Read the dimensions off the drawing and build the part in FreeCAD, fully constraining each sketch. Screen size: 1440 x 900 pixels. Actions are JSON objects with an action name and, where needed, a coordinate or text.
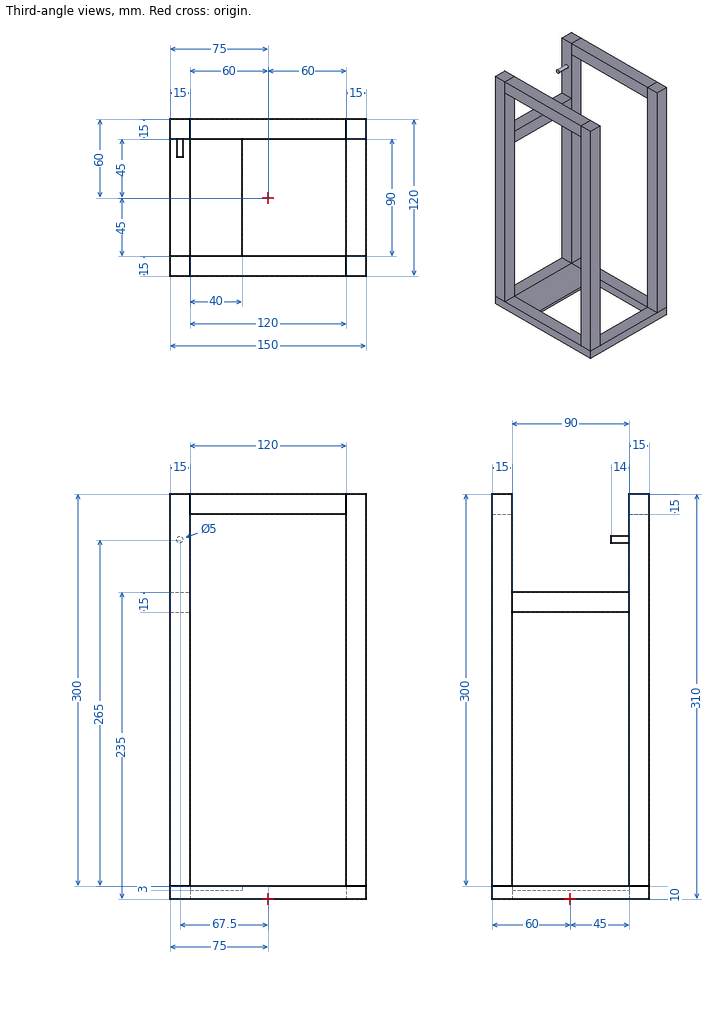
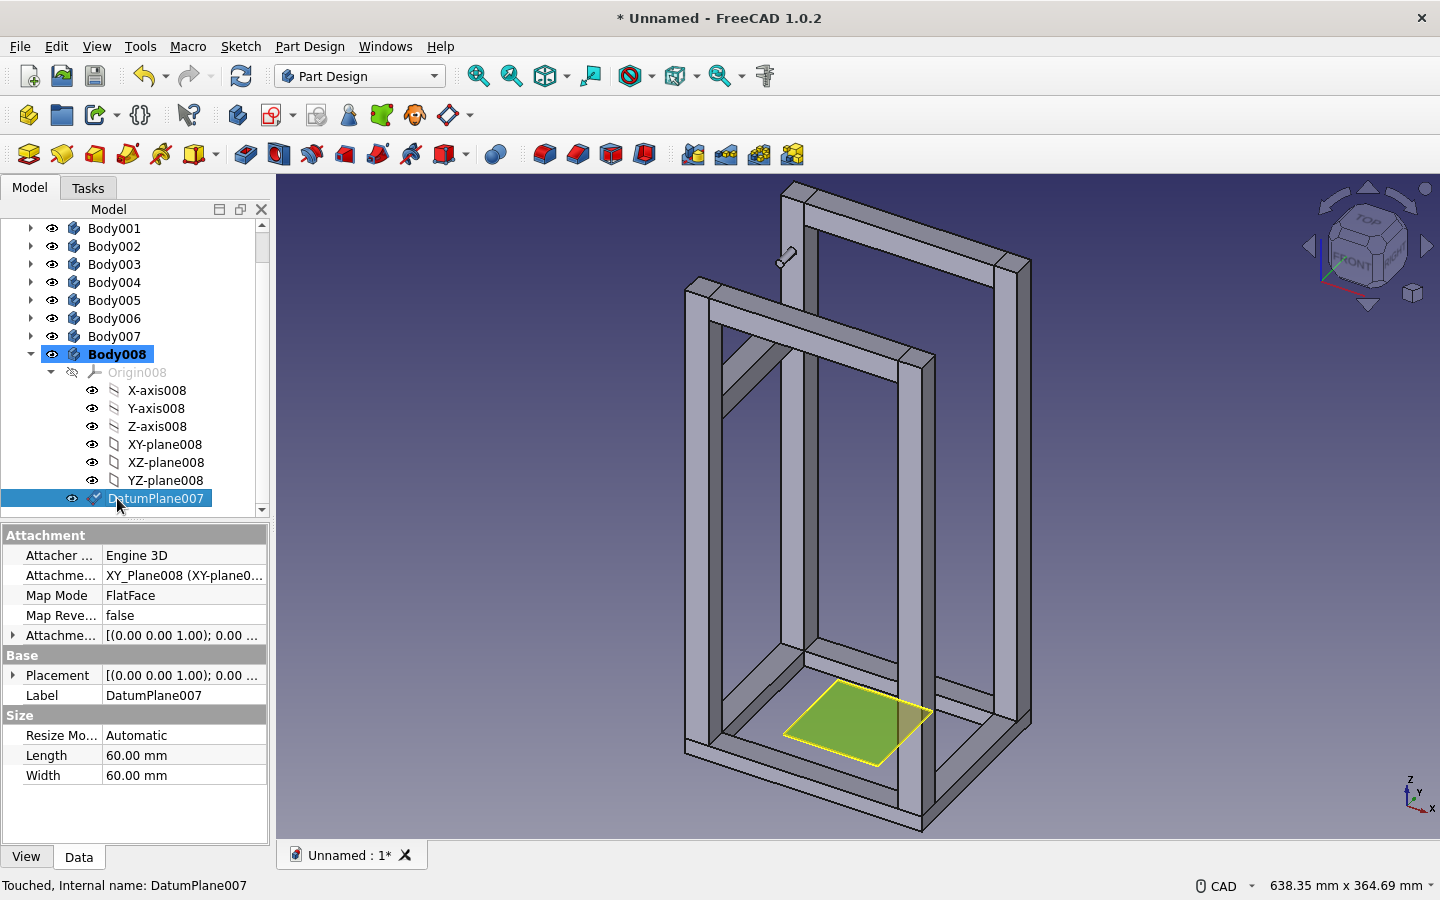
{"action": "left_click", "coordinate": [270, 116]}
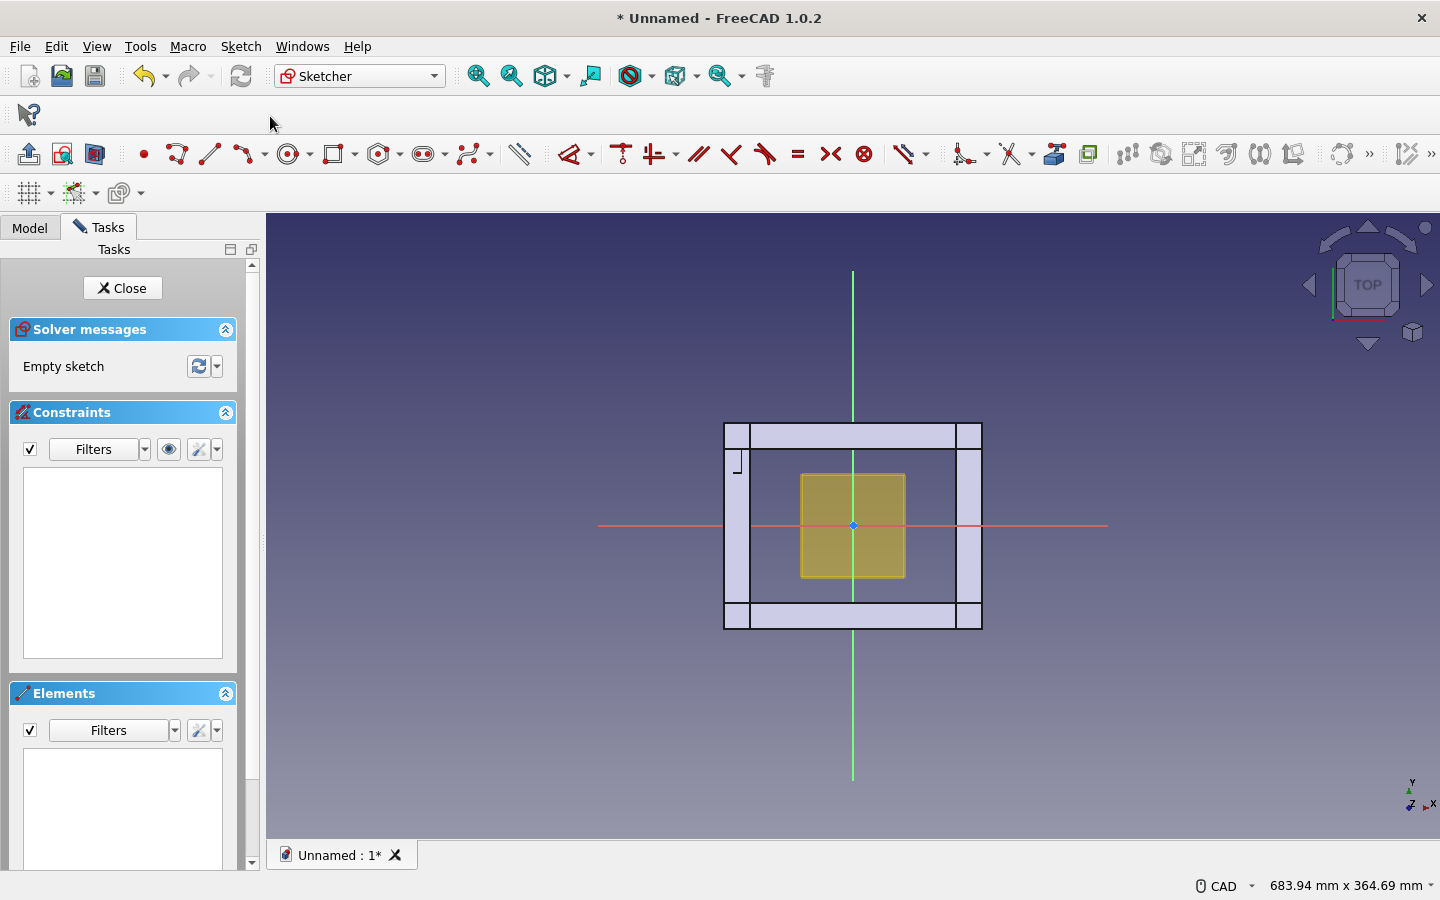
{"action": "scroll", "coordinate": [811, 526], "scroll_direction": "up", "scroll_amount": 5}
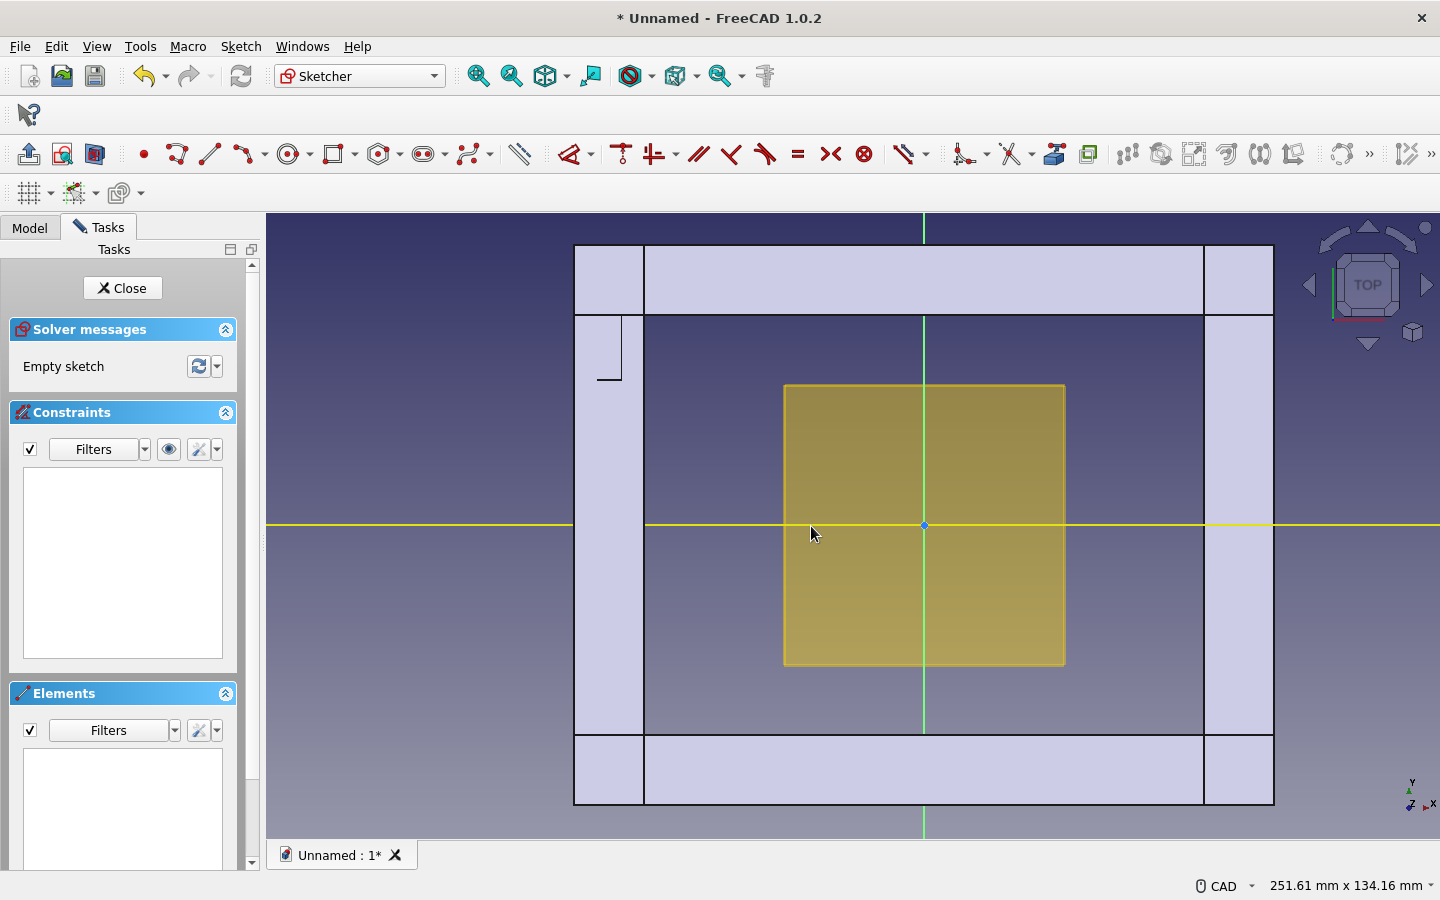
{"action": "left_click", "coordinate": [332, 154]}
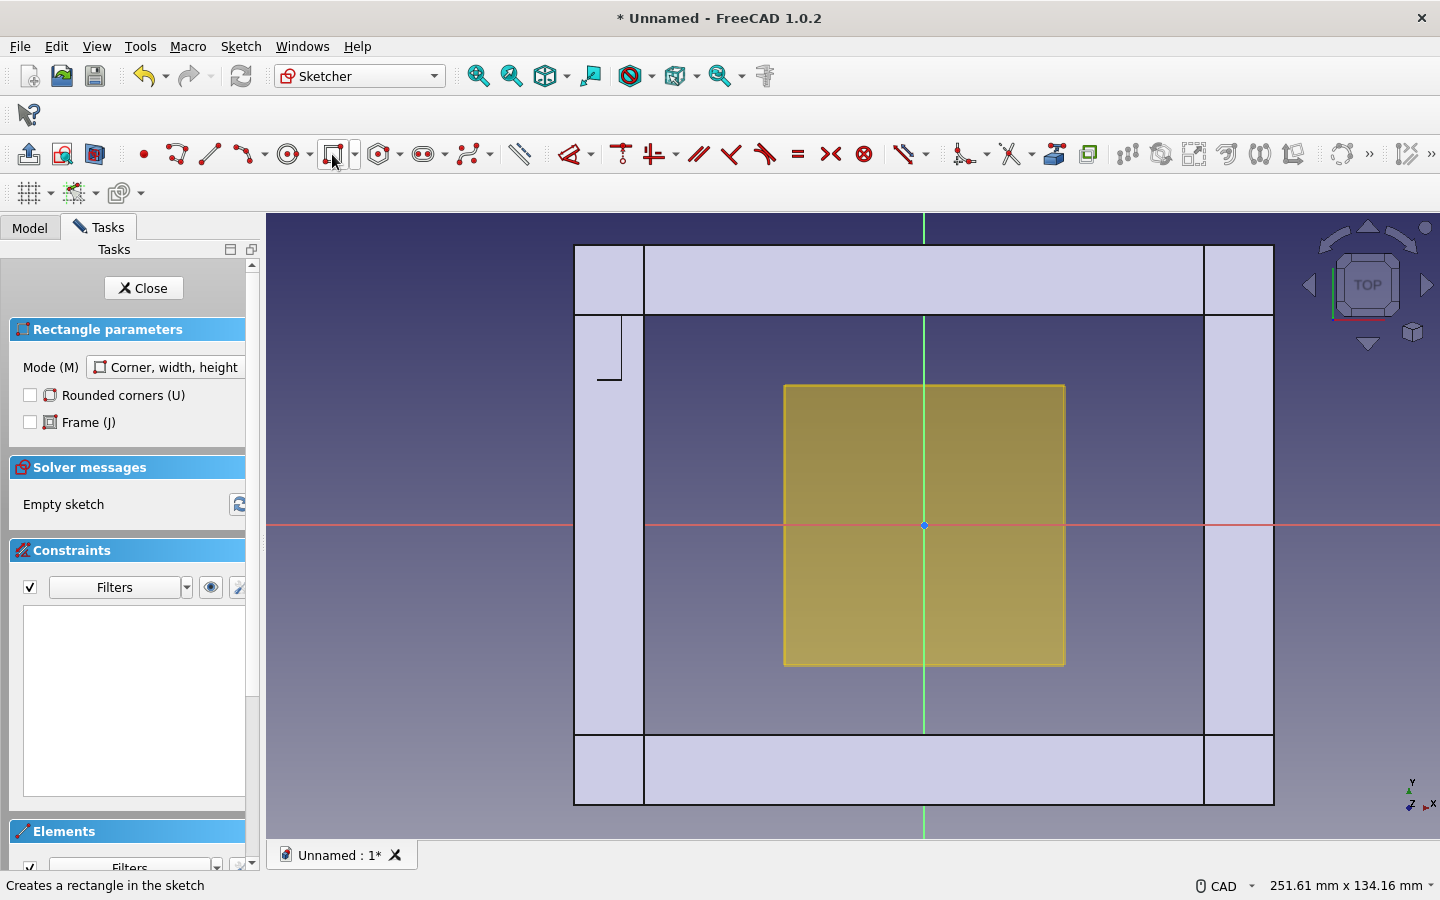
{"action": "left_click", "coordinate": [644, 315]}
{"action": "left_click", "coordinate": [831, 735]}
{"action": "key", "text": "Escape"}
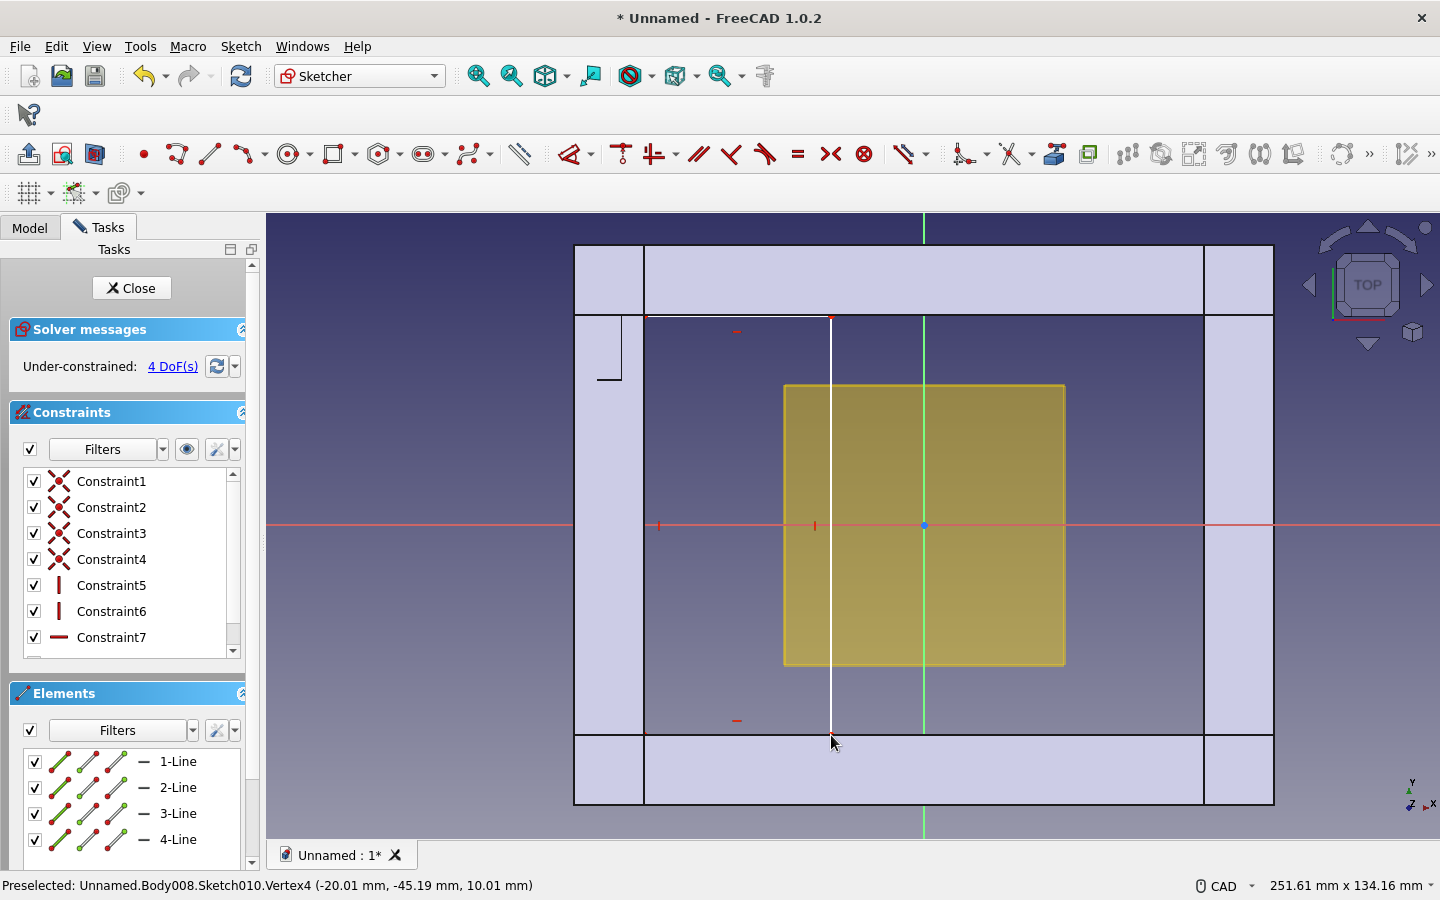
{"action": "left_click", "coordinate": [568, 154]}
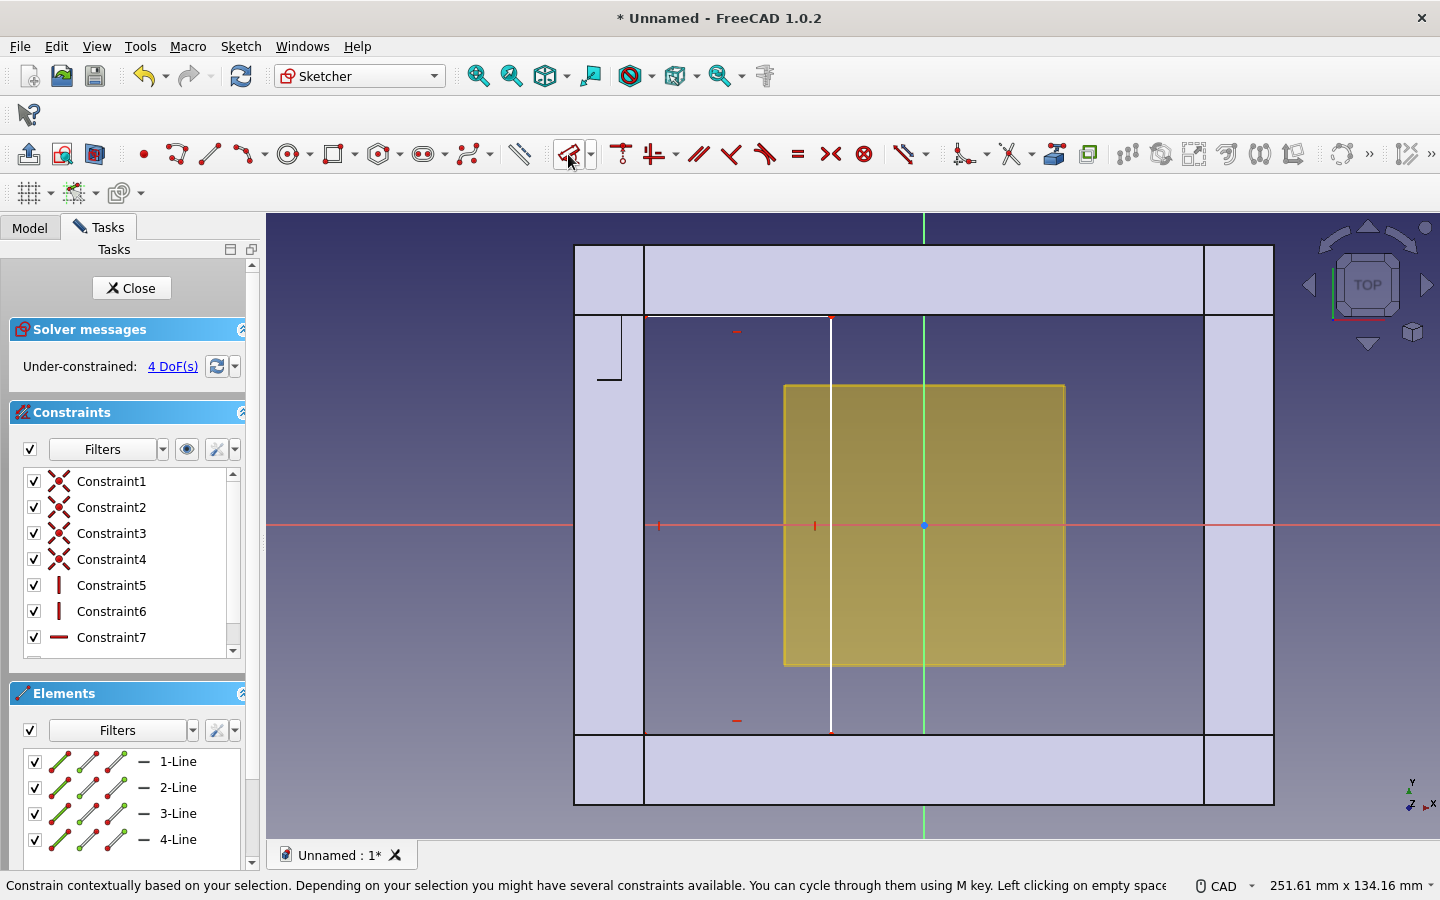
{"action": "left_click", "coordinate": [644, 442]}
{"action": "left_click", "coordinate": [610, 429]}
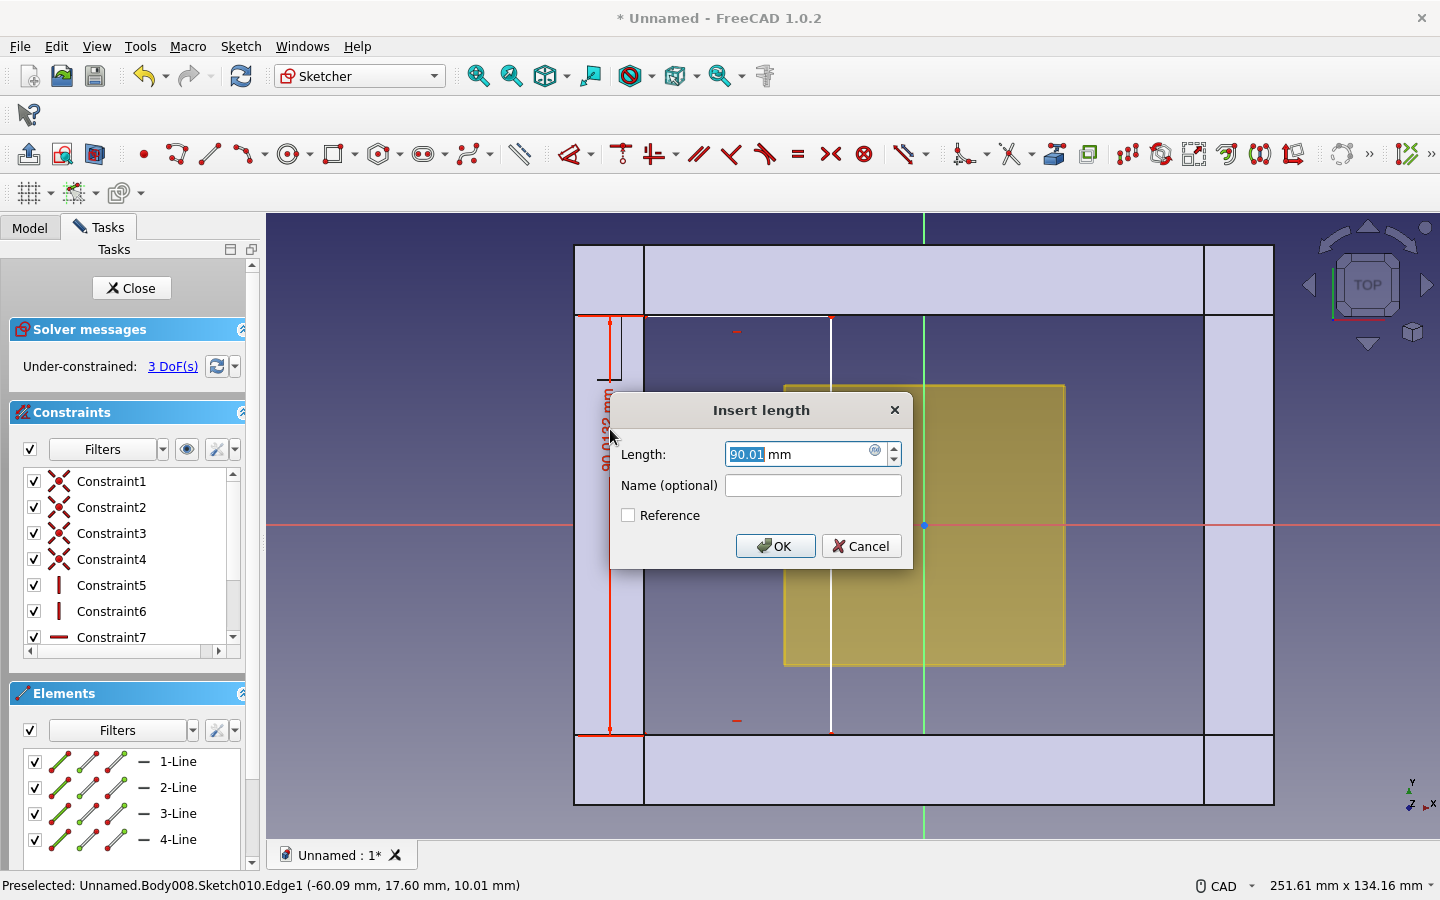
{"action": "type", "text": "90"}
{"action": "key", "text": "Return"}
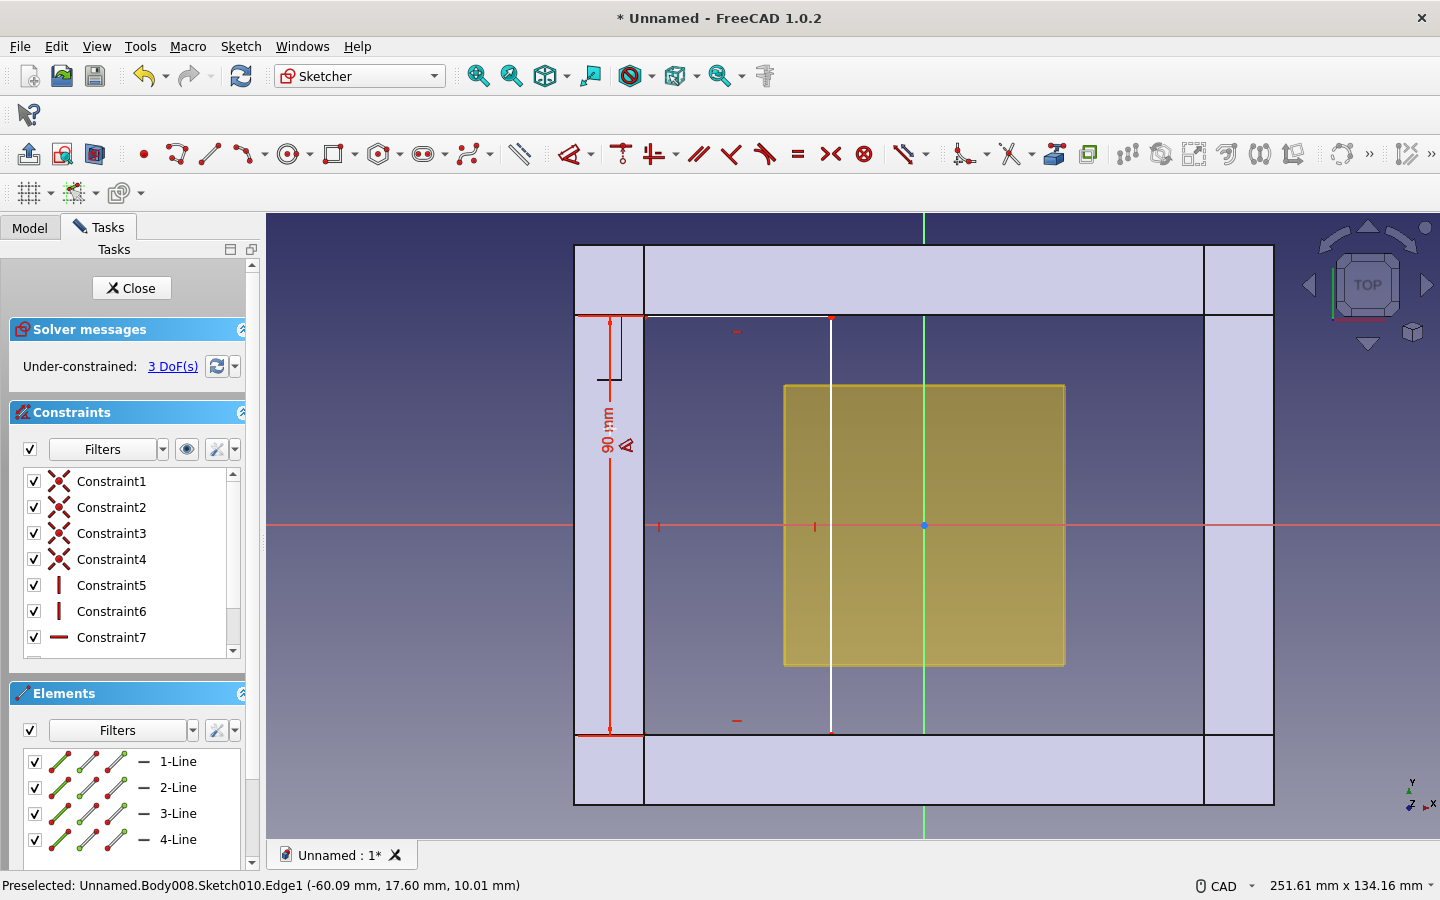
{"action": "left_click", "coordinate": [700, 736]}
{"action": "left_click", "coordinate": [738, 770]}